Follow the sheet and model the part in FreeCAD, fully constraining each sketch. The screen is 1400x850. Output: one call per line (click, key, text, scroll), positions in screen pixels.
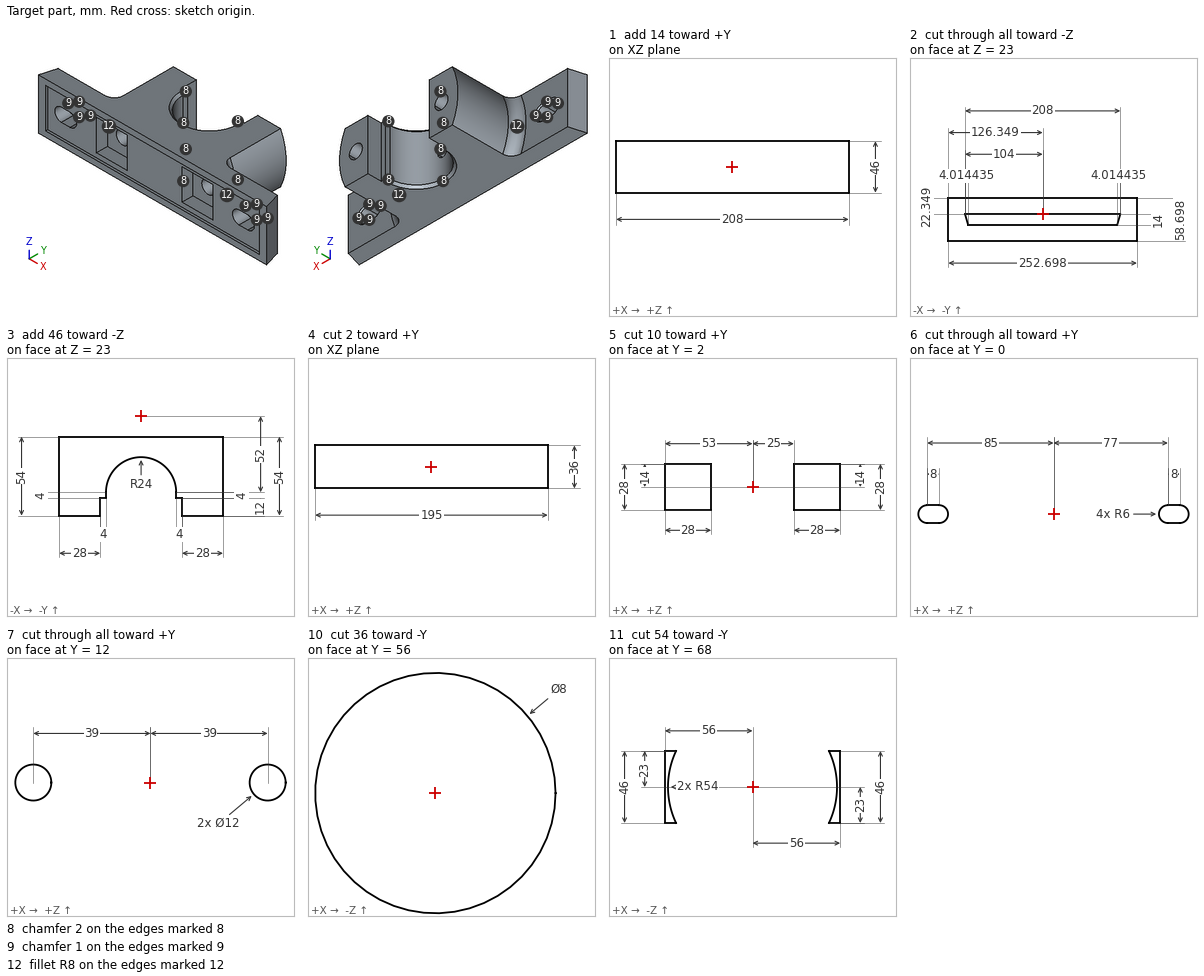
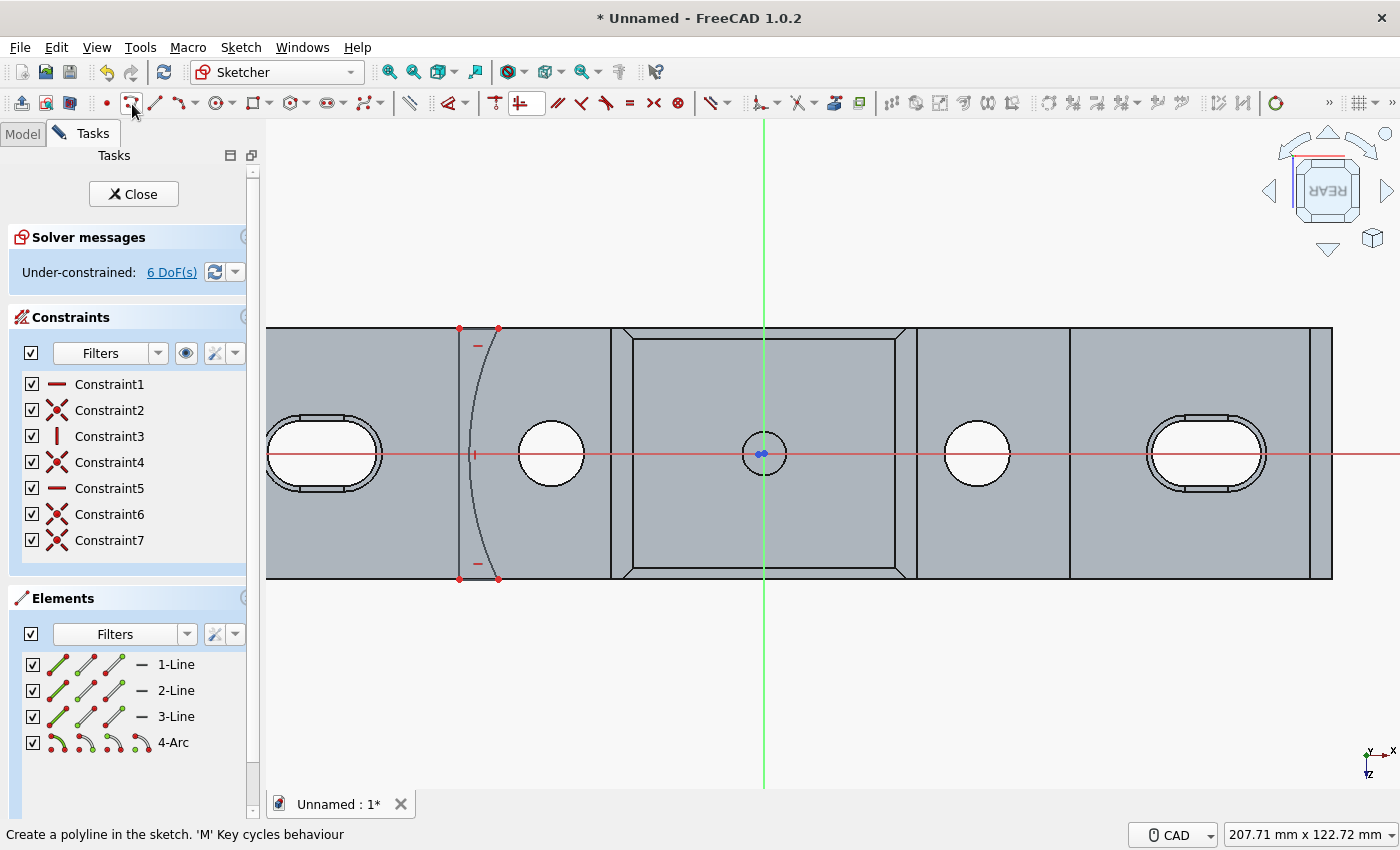
click(1031, 579)
click(1070, 579)
click(1070, 328)
click(1031, 328)
right_click(1031, 328)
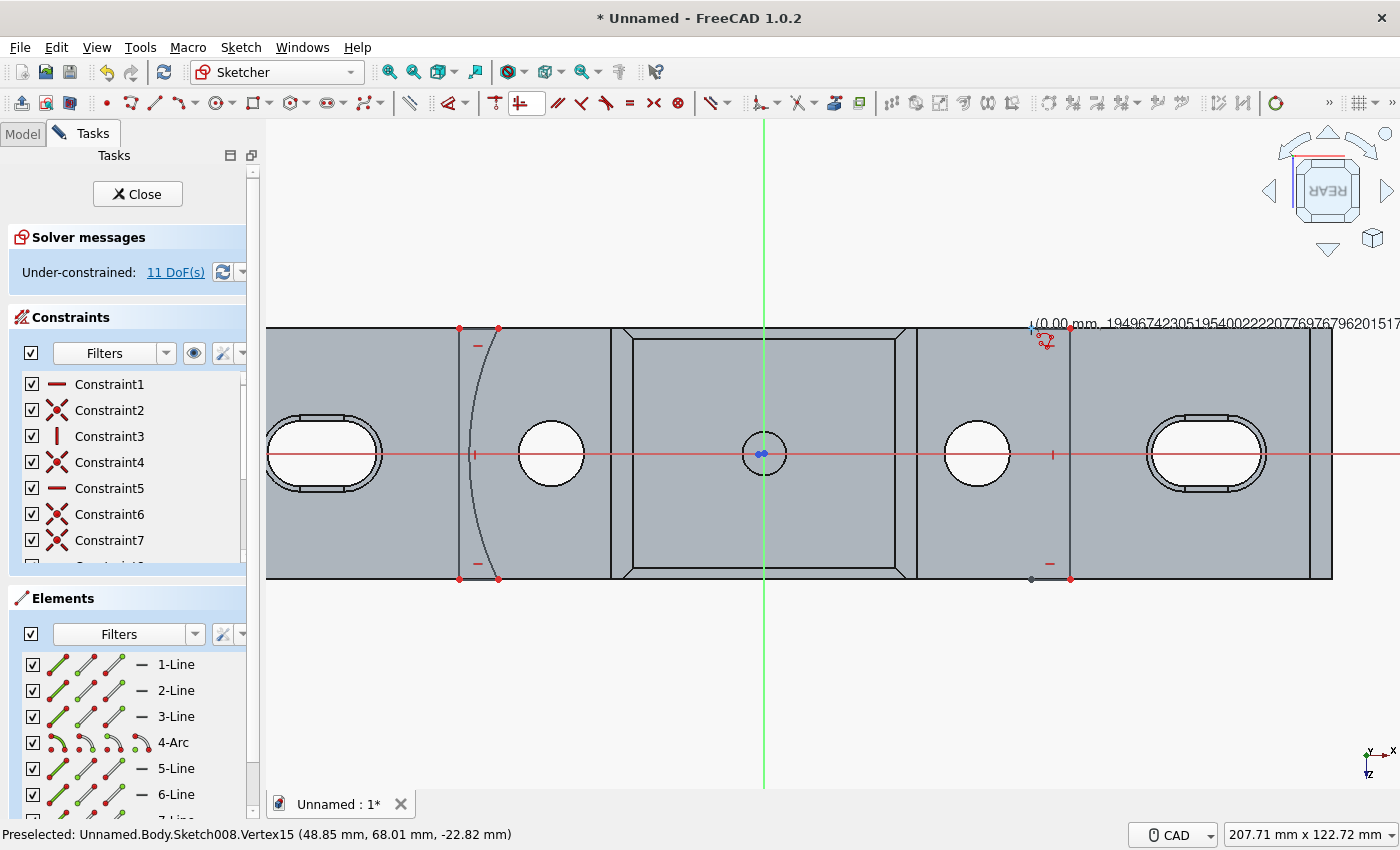
key(g)
key(3)
key(a)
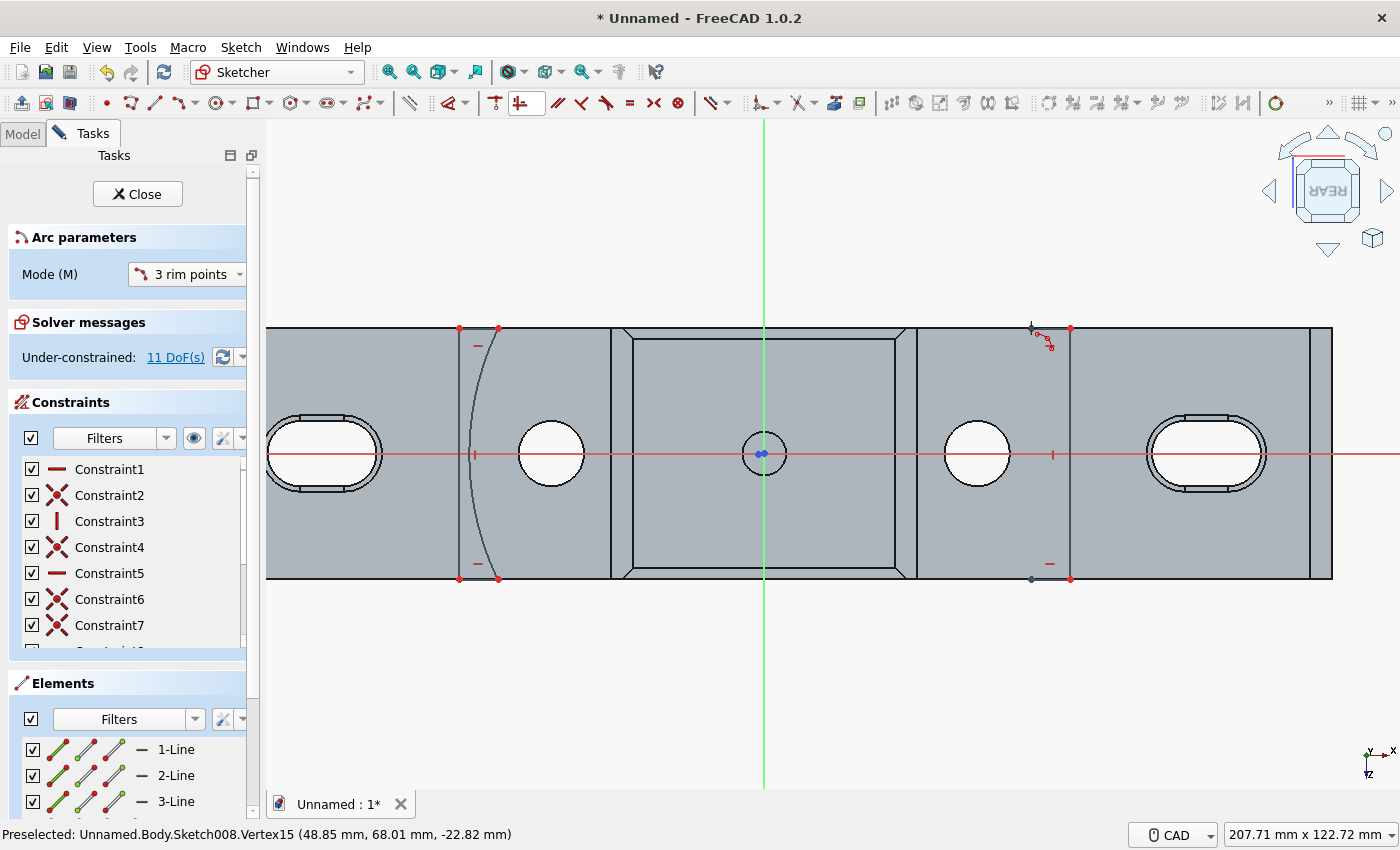
click(1031, 329)
click(1031, 580)
click(1055, 505)
key(Escape)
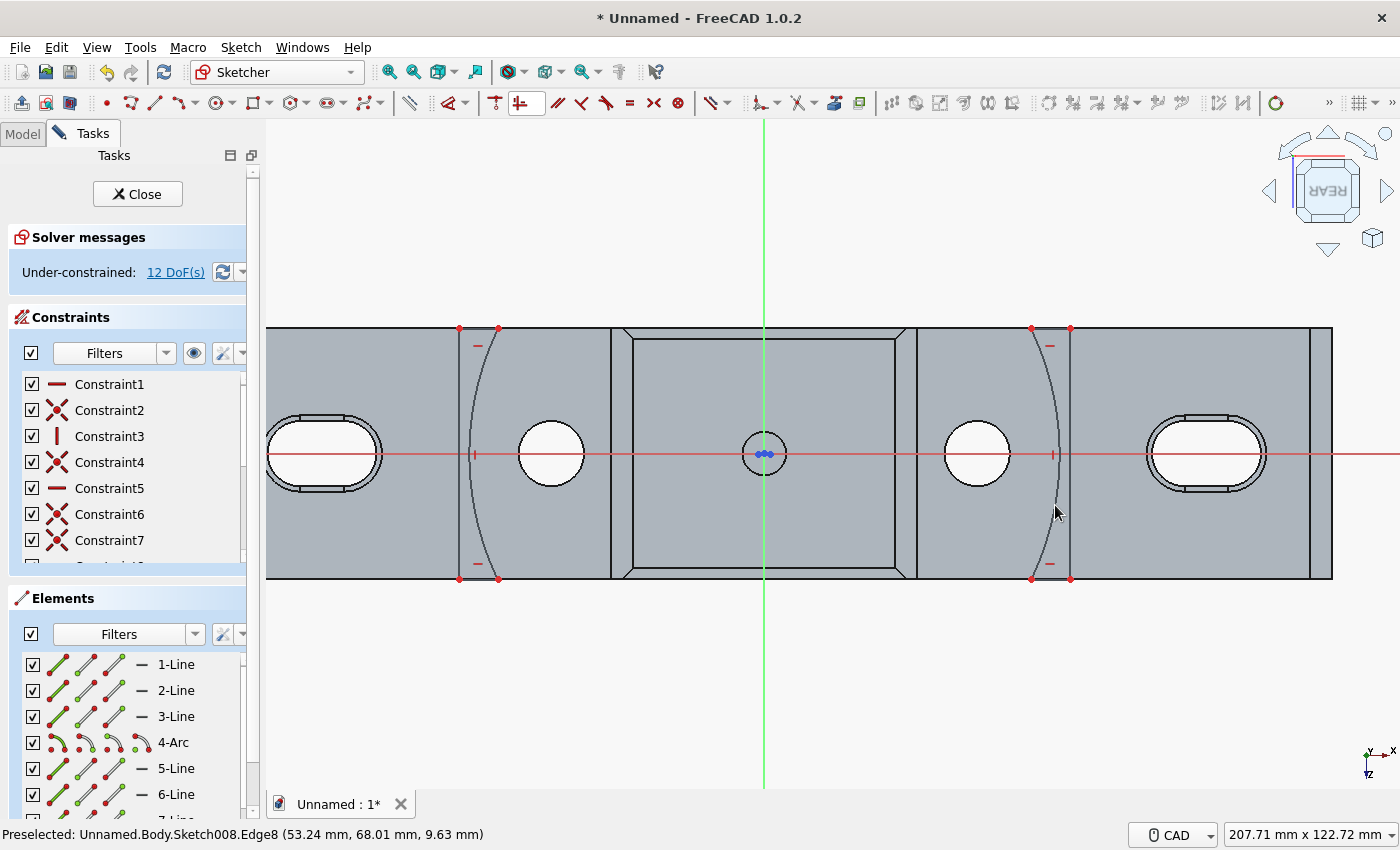
click(474, 403)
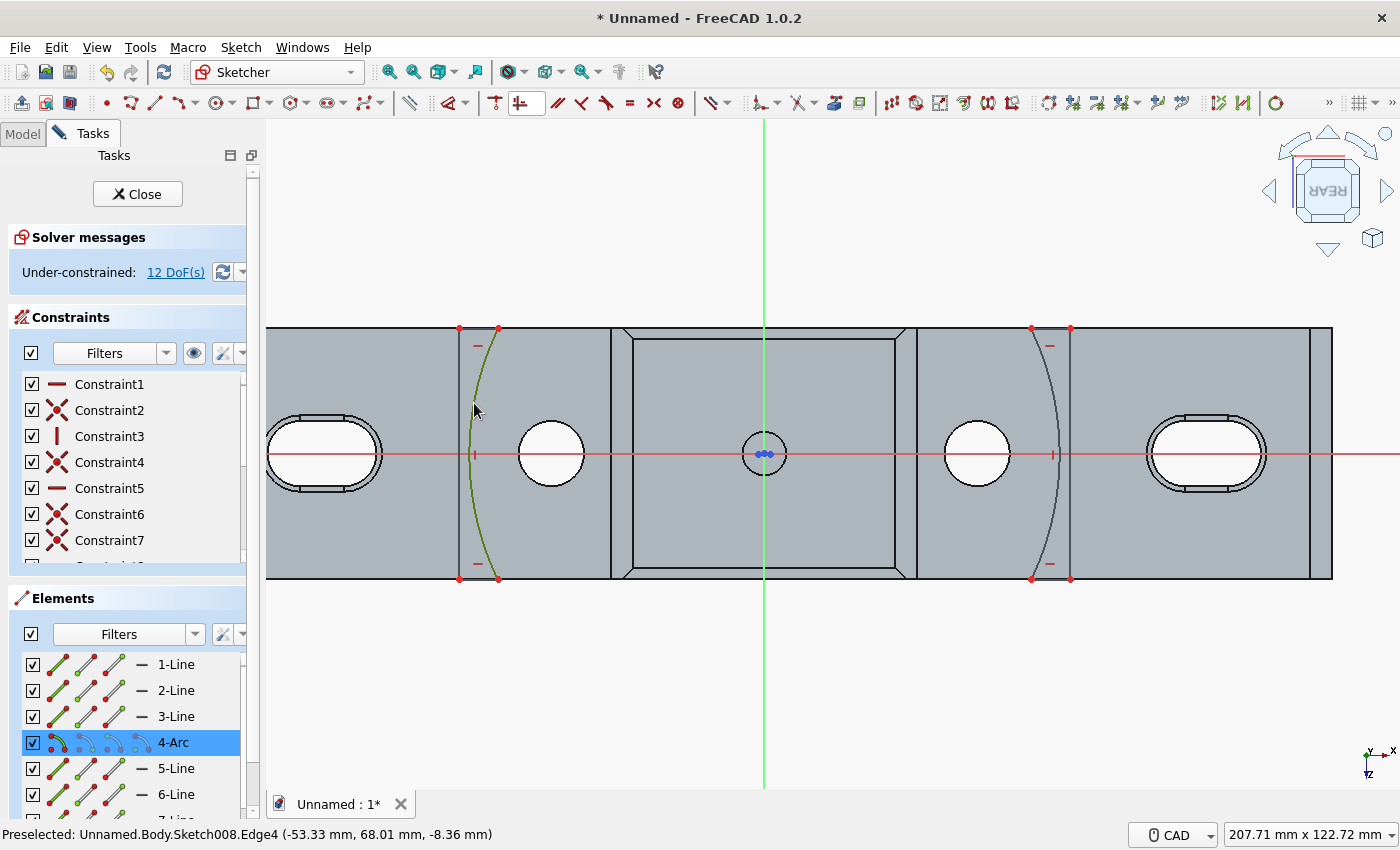
click(1055, 506)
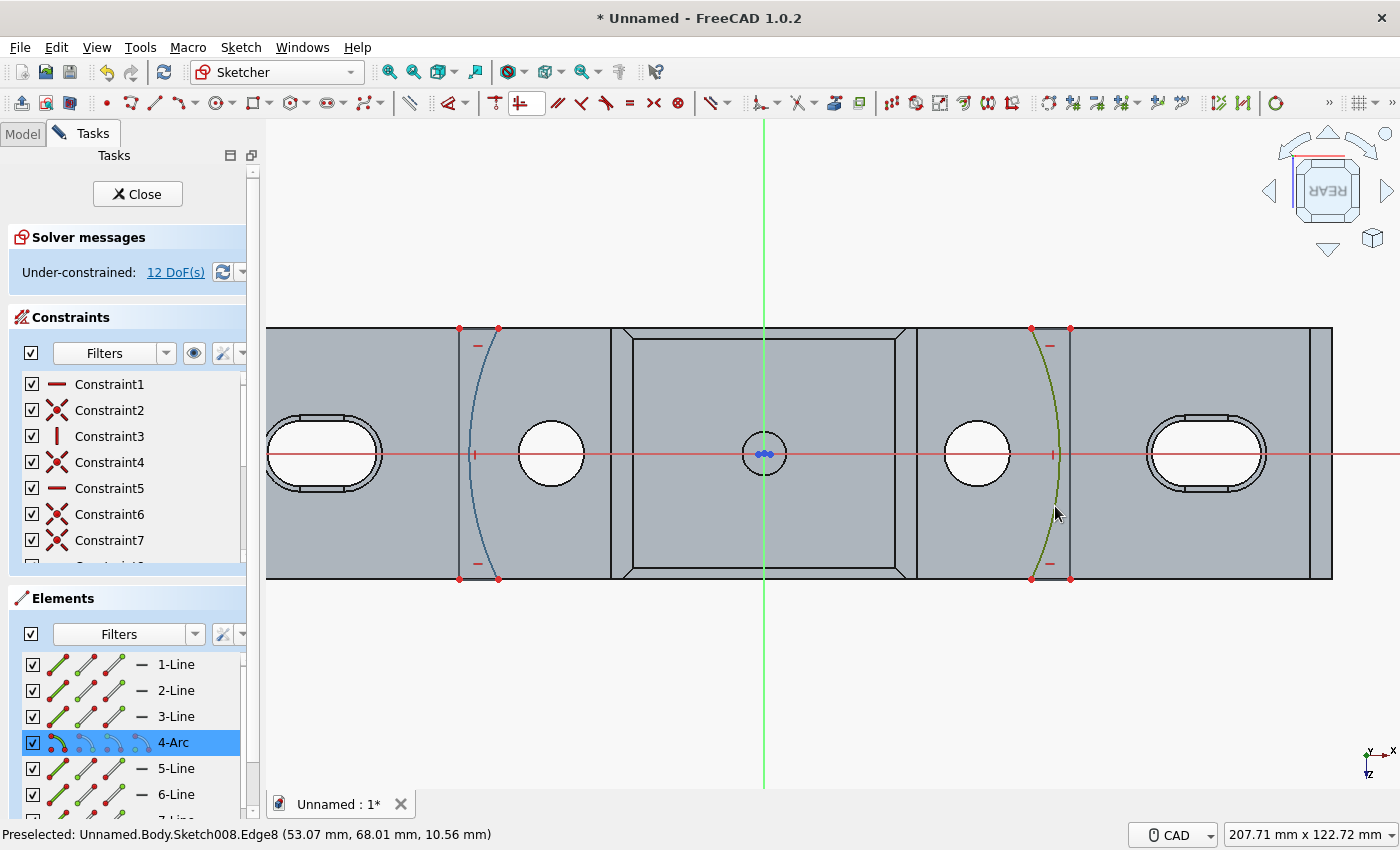
key(c)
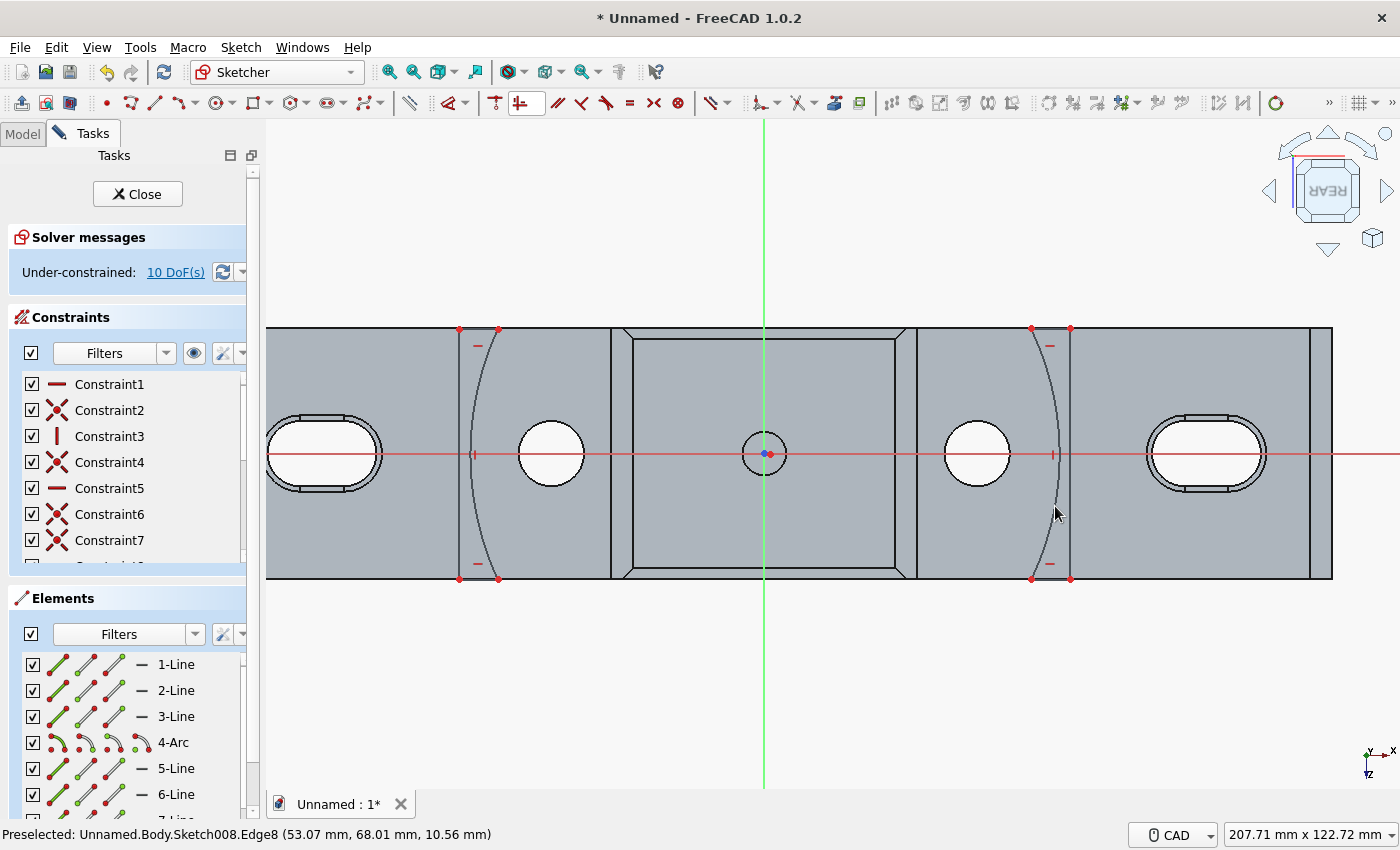
drag(754, 444, 780, 464)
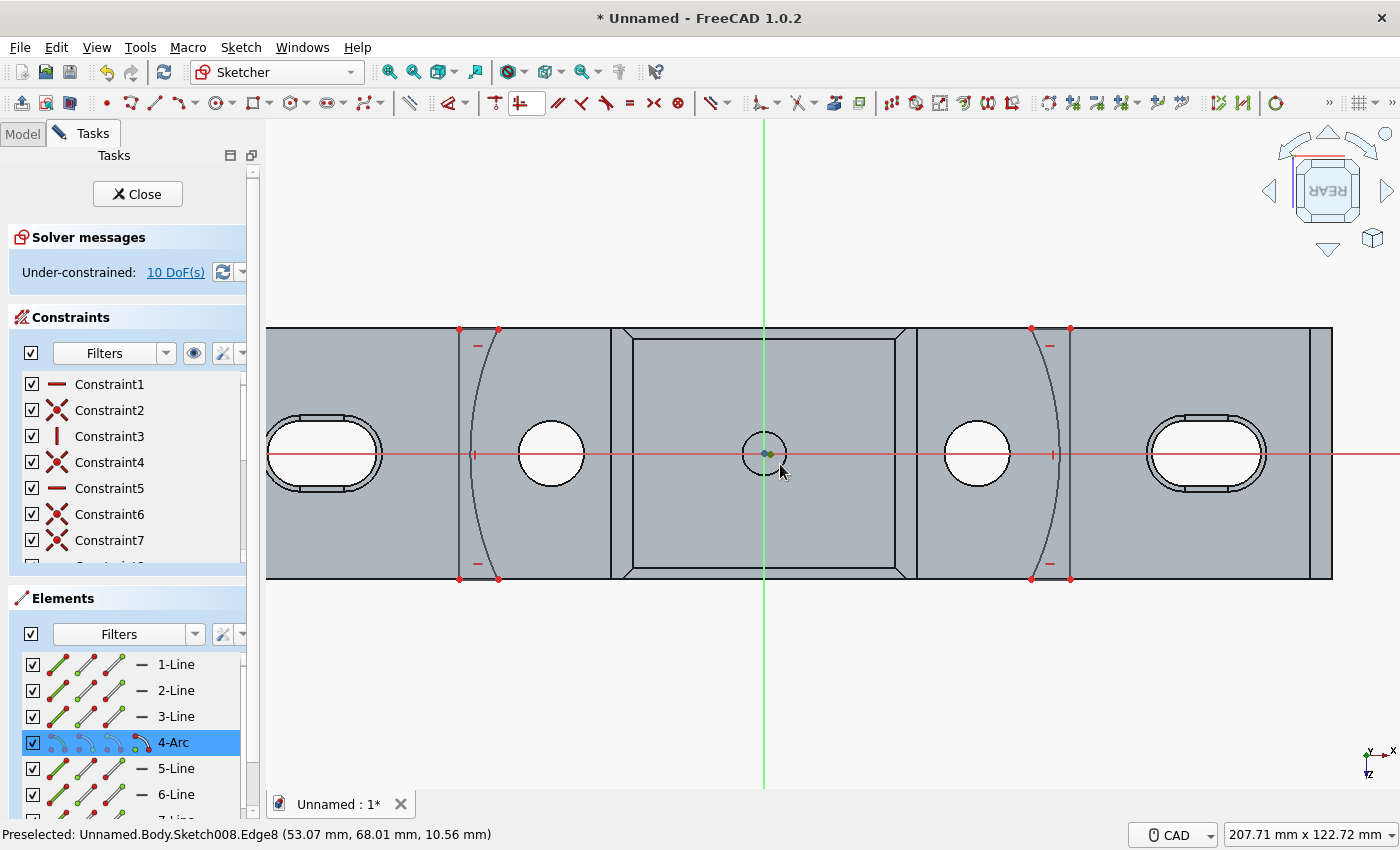
key(c)